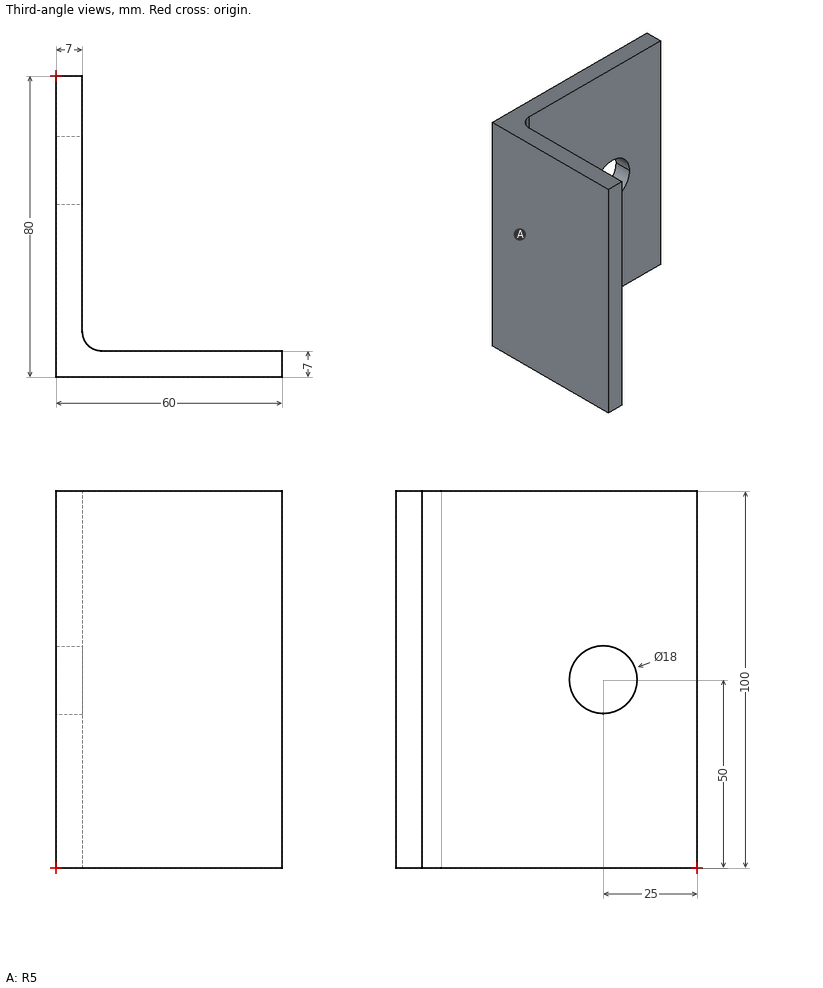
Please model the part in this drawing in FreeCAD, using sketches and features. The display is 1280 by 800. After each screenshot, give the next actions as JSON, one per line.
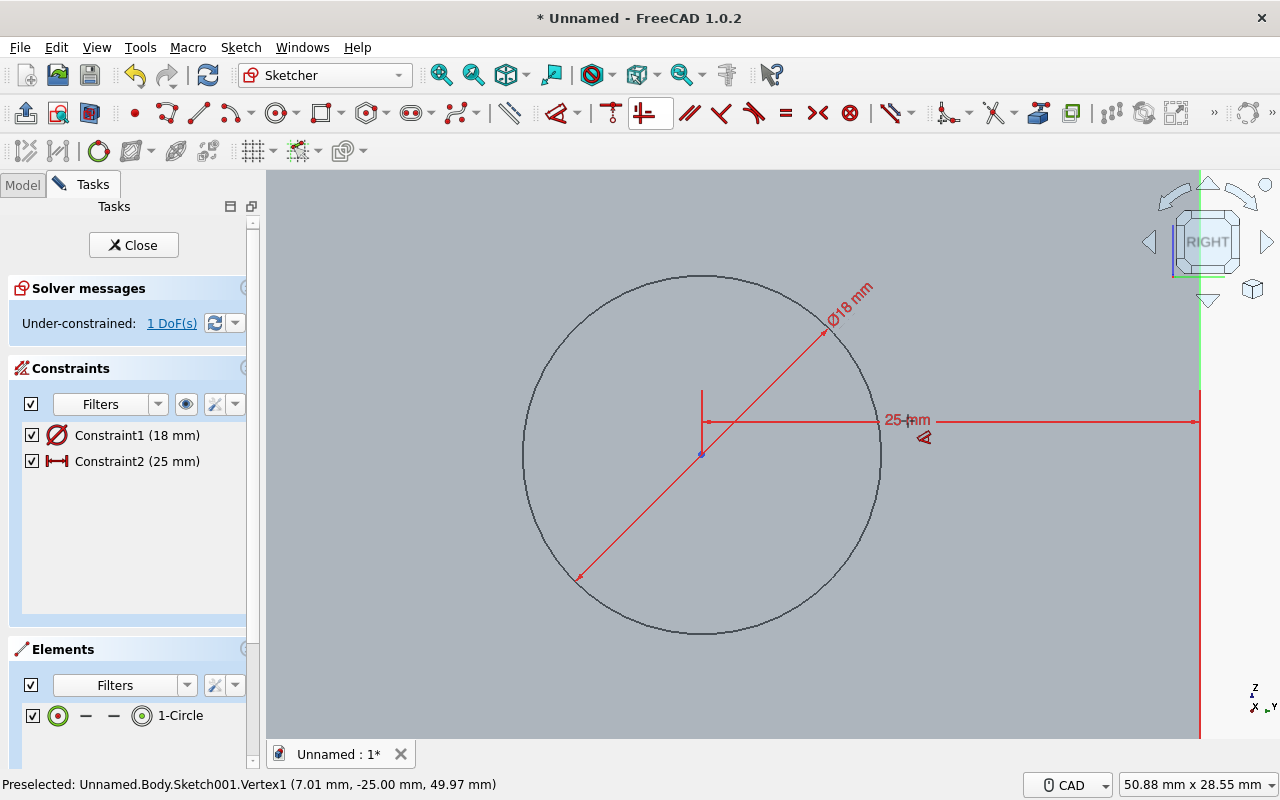
{"action": "left_click", "coordinate": [702, 455]}
{"action": "left_click", "coordinate": [668, 583]}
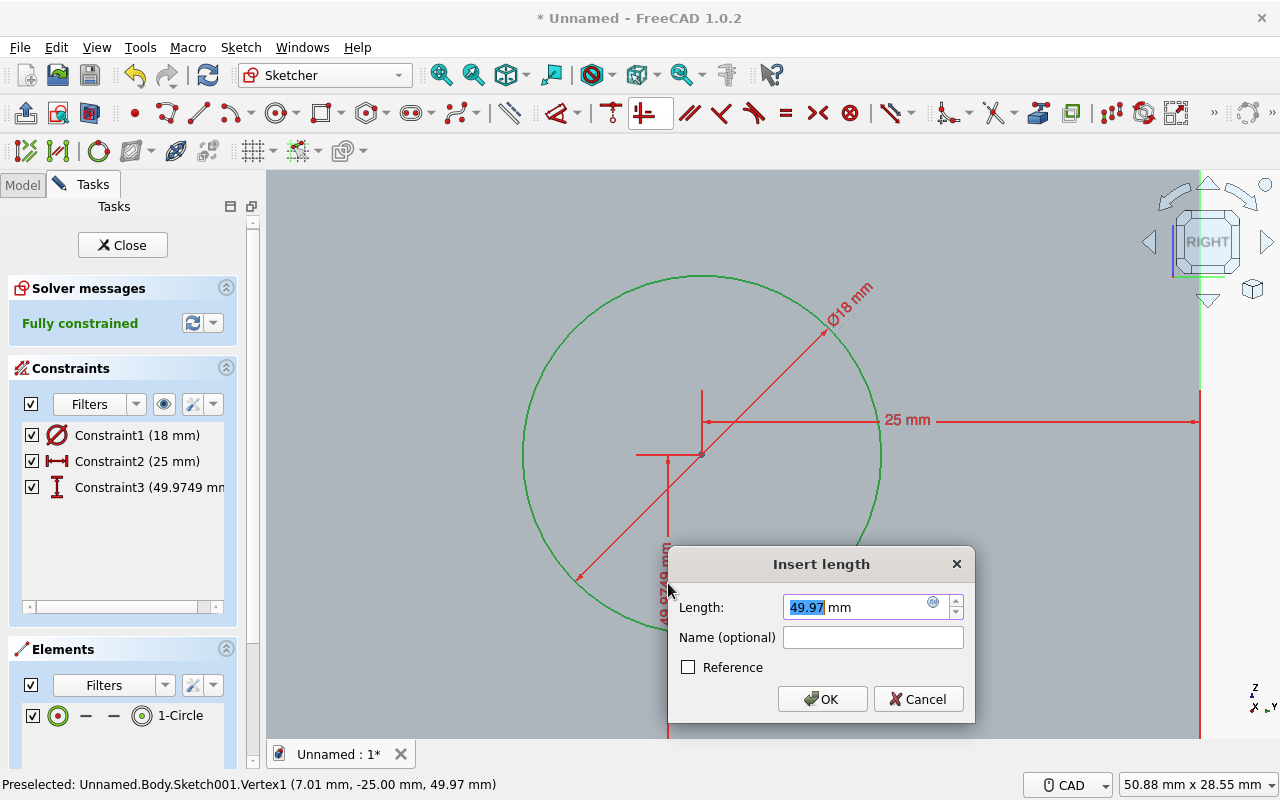
{"action": "type", "text": "50"}
{"action": "key", "text": "Return"}
{"action": "key", "text": "Escape"}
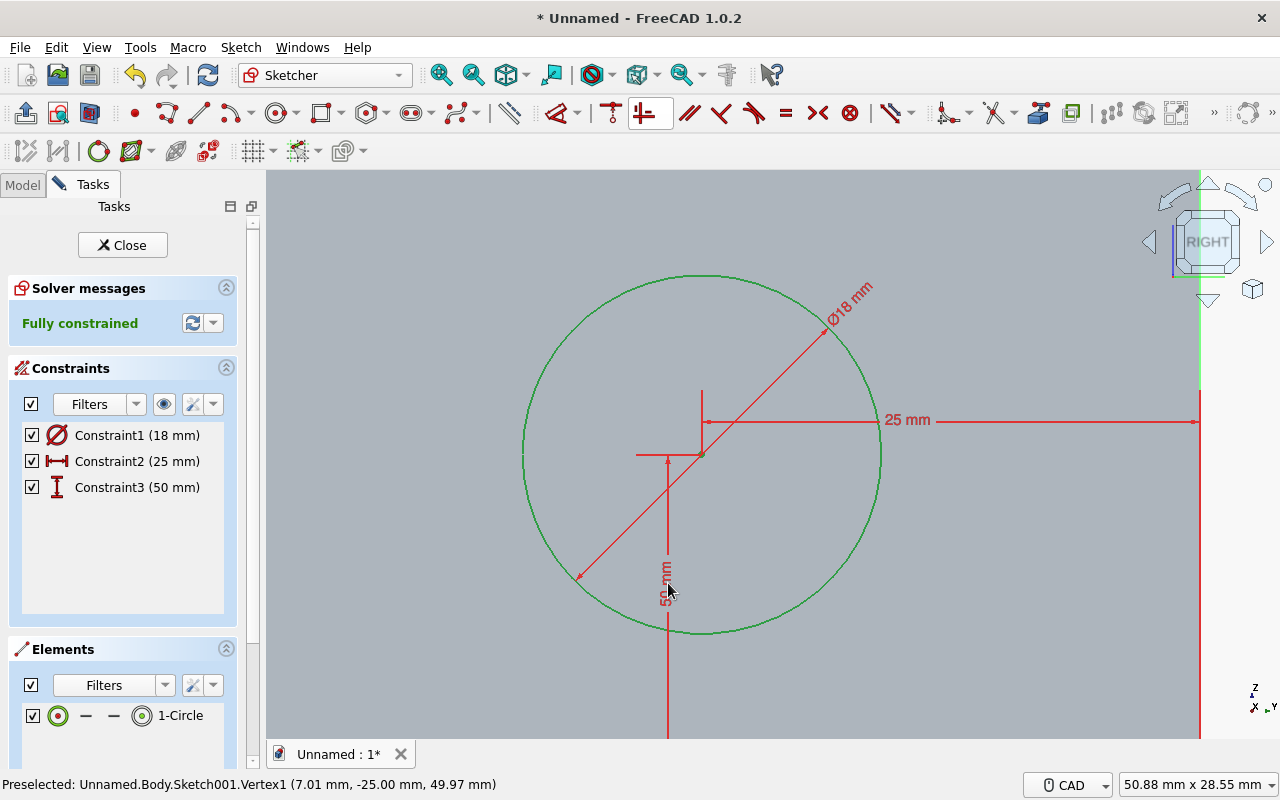
{"action": "left_click", "coordinate": [123, 245]}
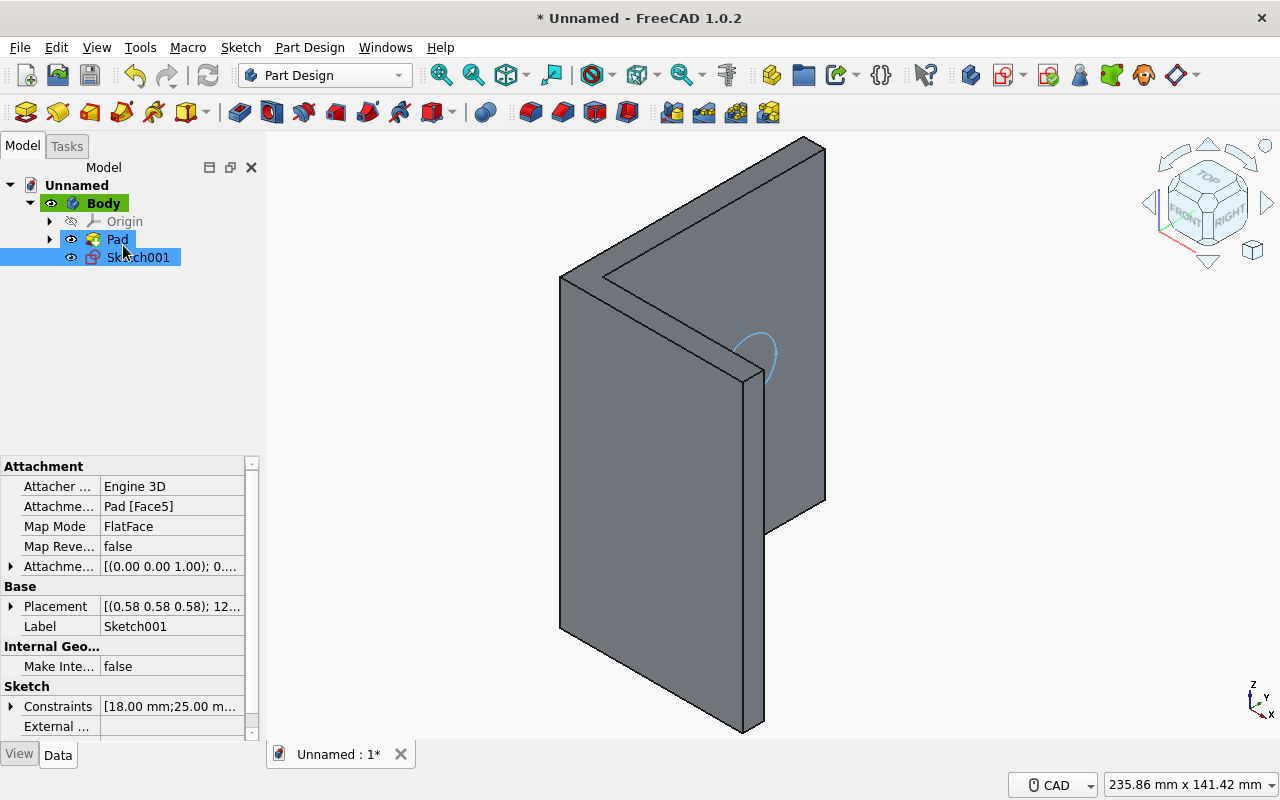
{"action": "left_click", "coordinate": [240, 112]}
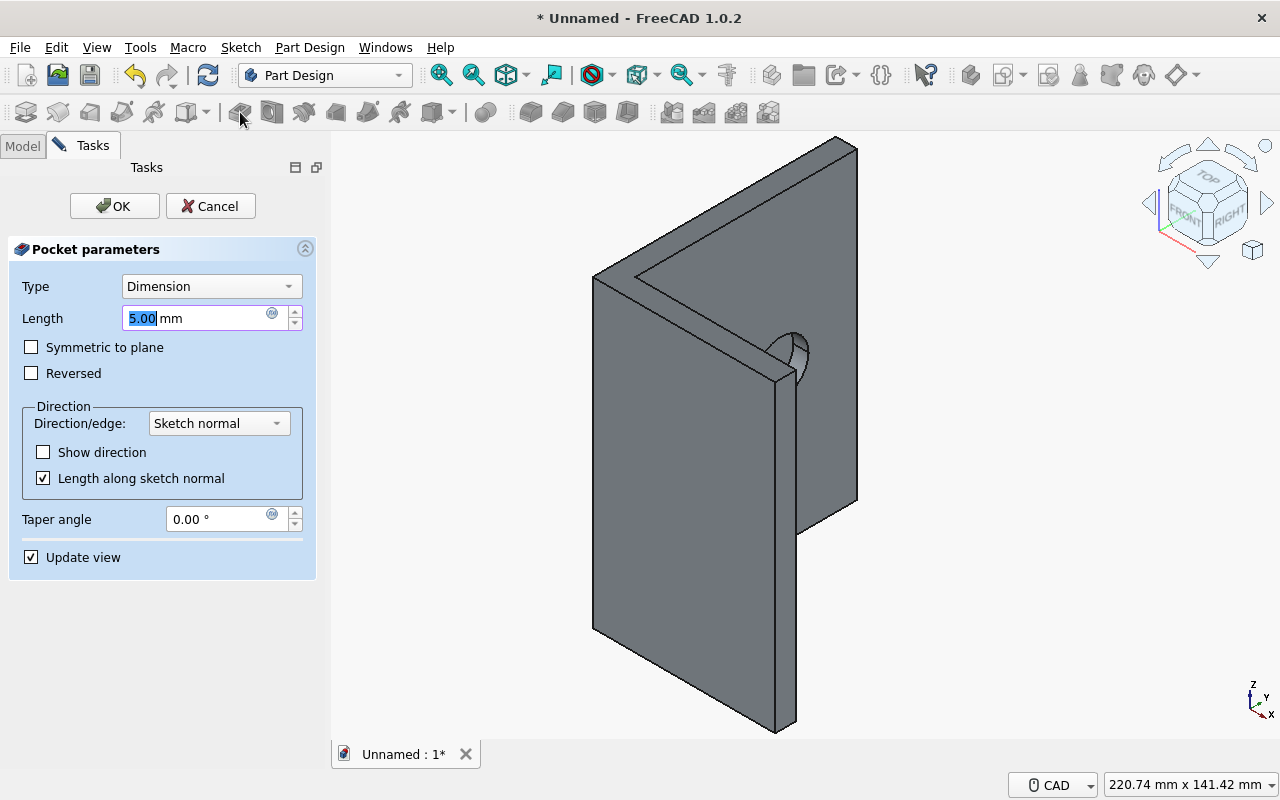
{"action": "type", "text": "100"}
{"action": "key", "text": "Tab"}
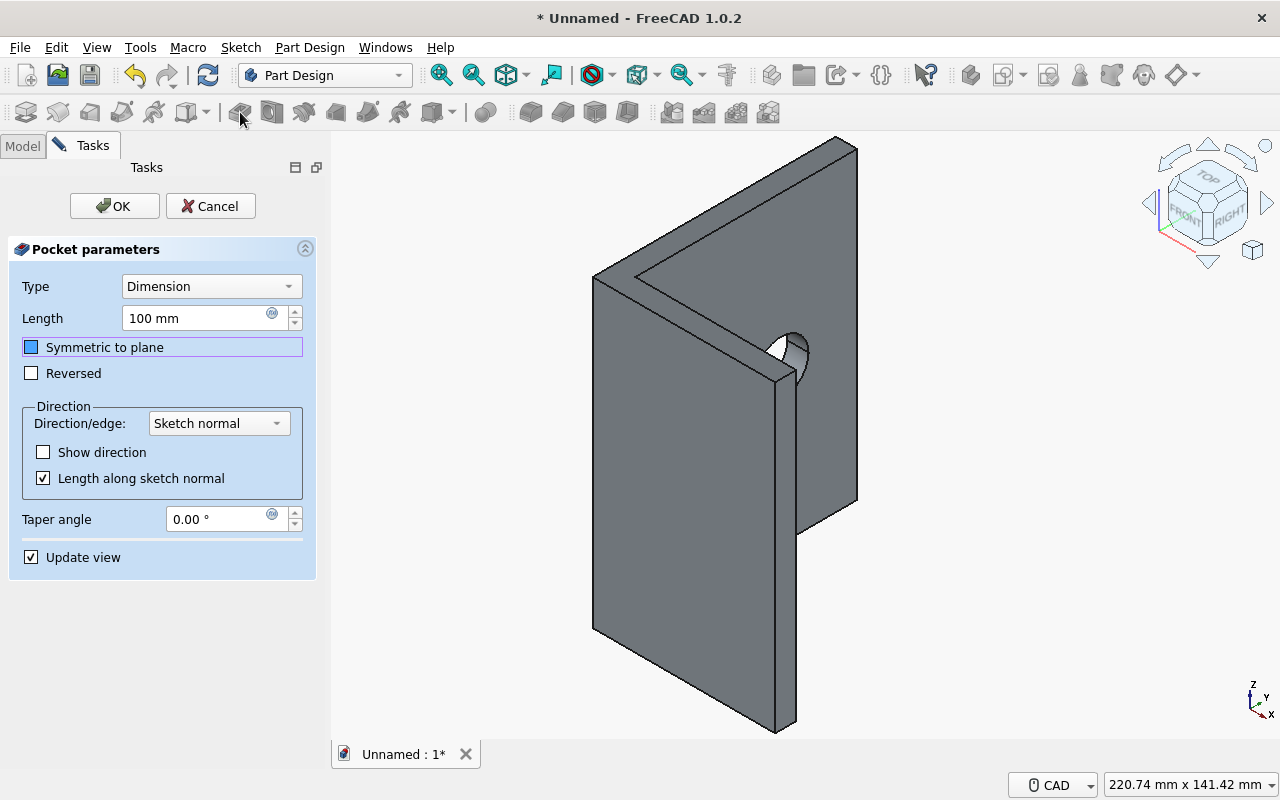
{"action": "left_click", "coordinate": [115, 206]}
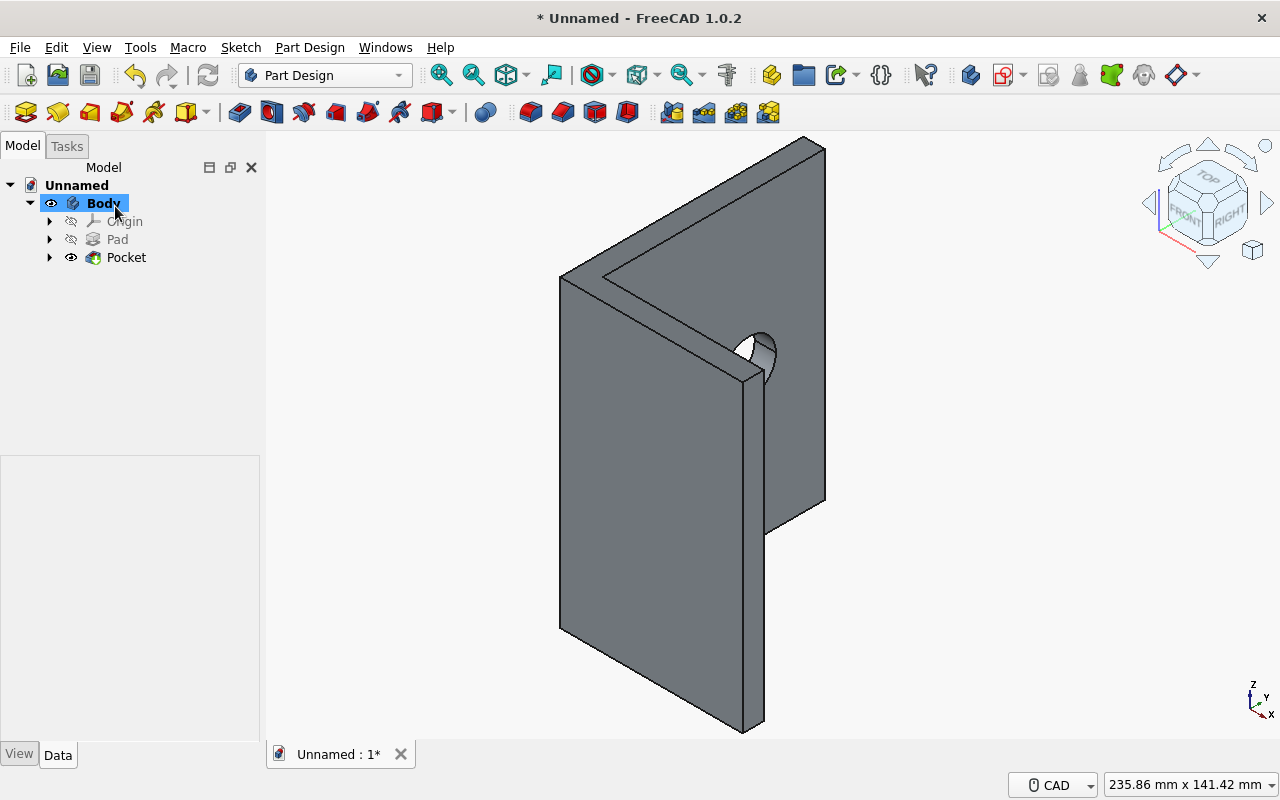
{"action": "key", "text": "2"}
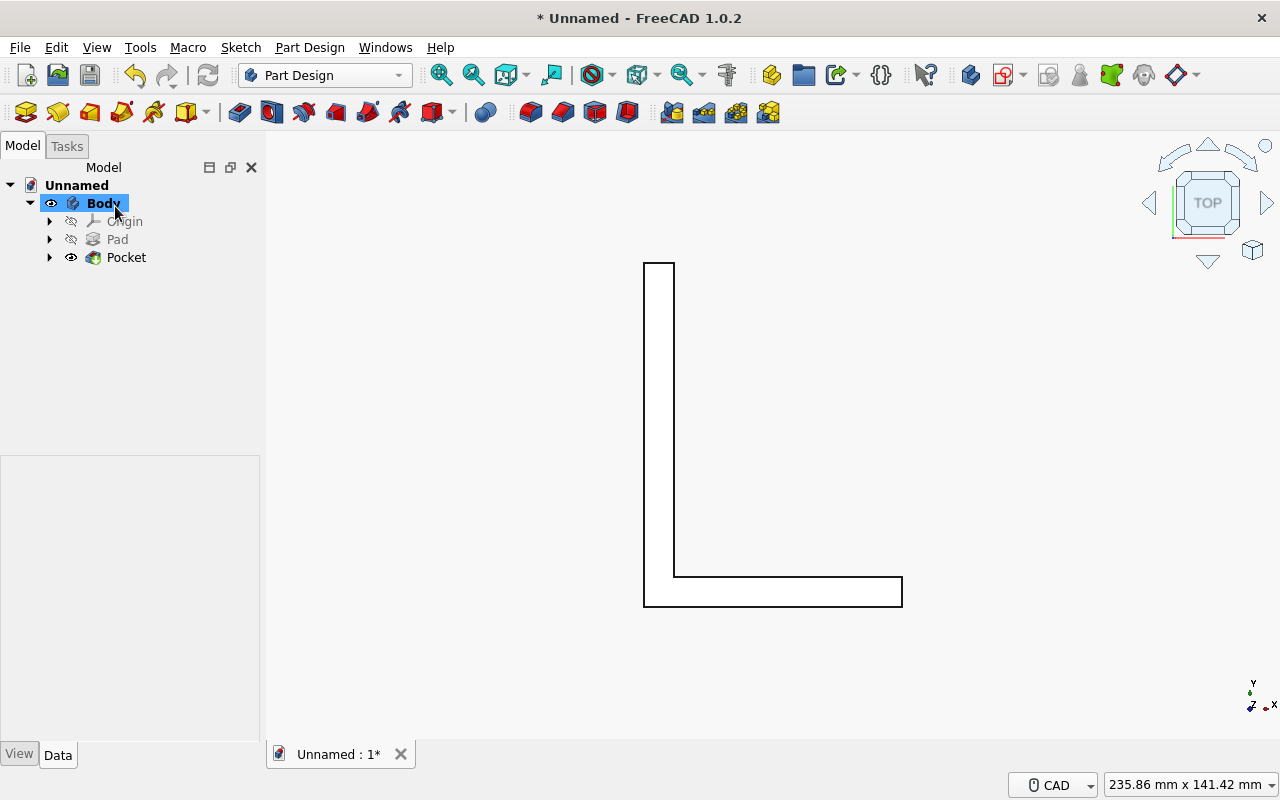
{"action": "key", "text": "0"}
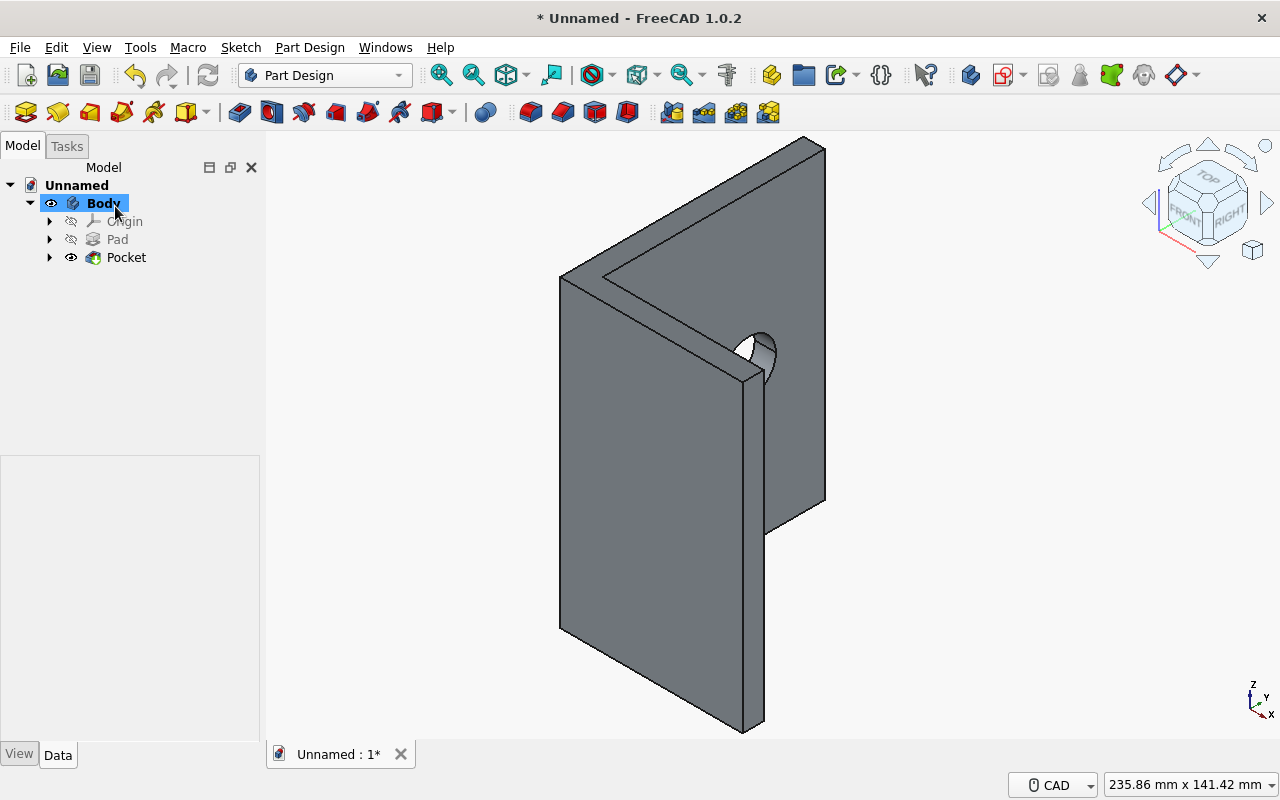
{"action": "key", "text": "1"}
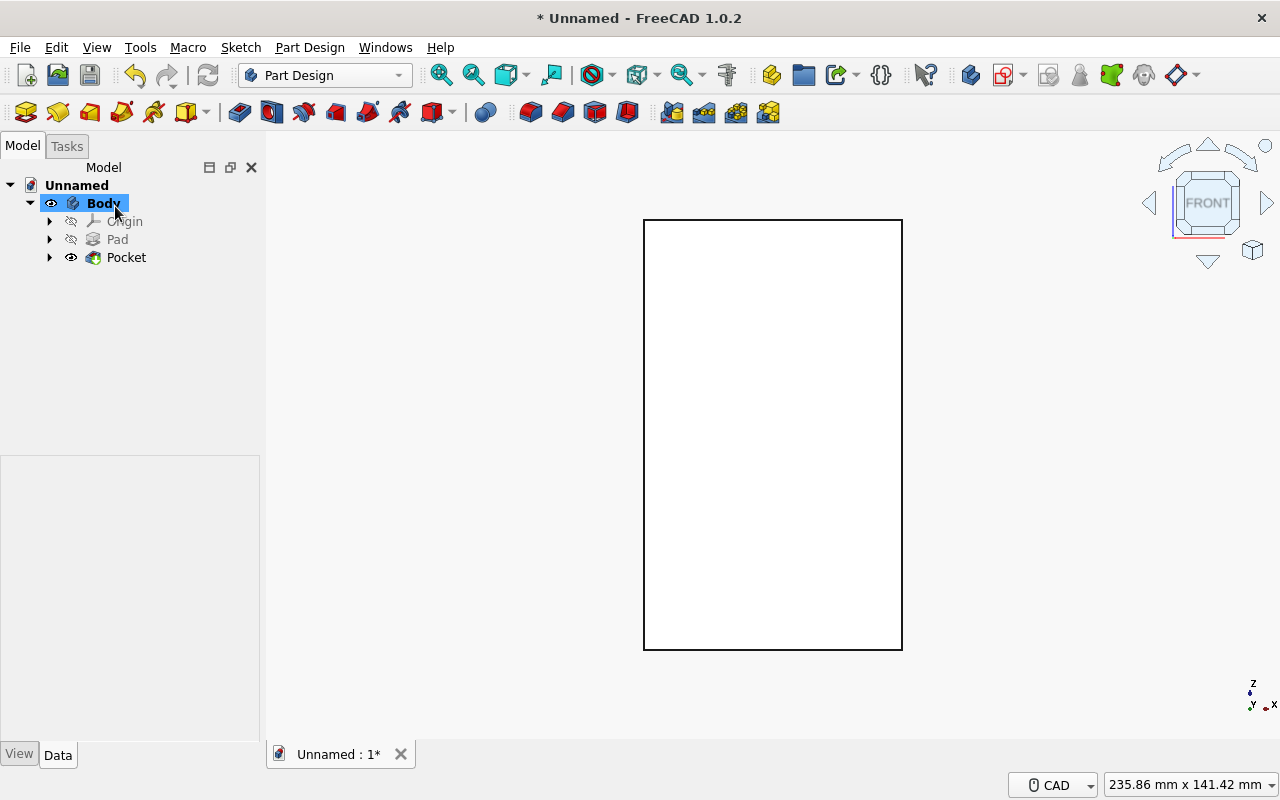
{"action": "key", "text": "3"}